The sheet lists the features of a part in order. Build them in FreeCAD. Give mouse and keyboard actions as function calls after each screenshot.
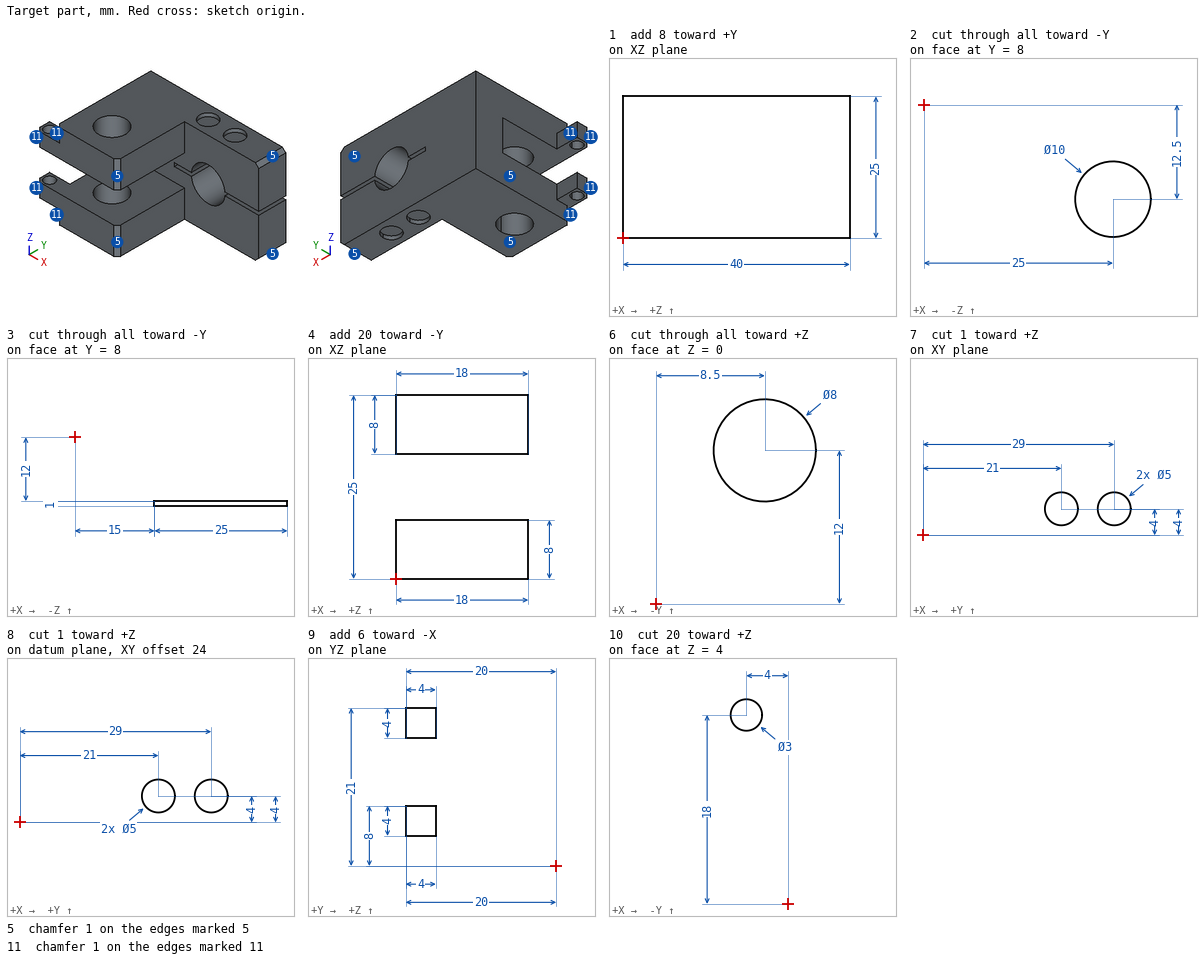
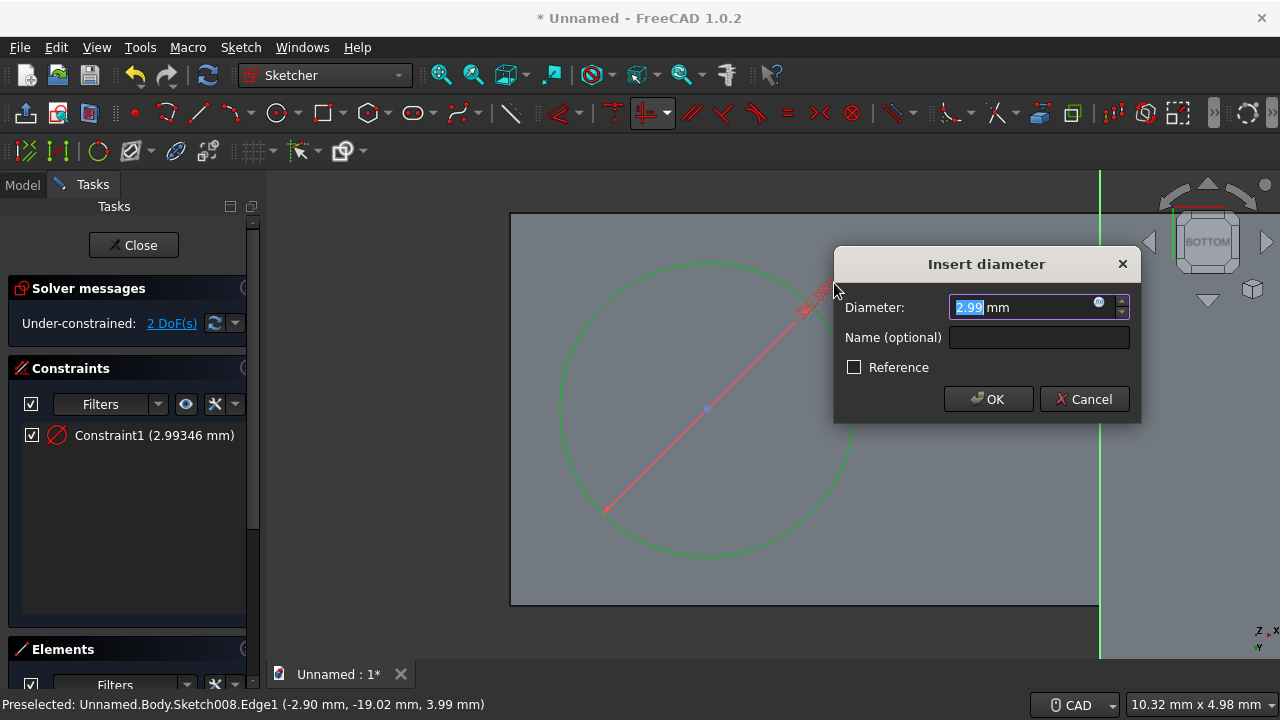
text(3)
key(Return)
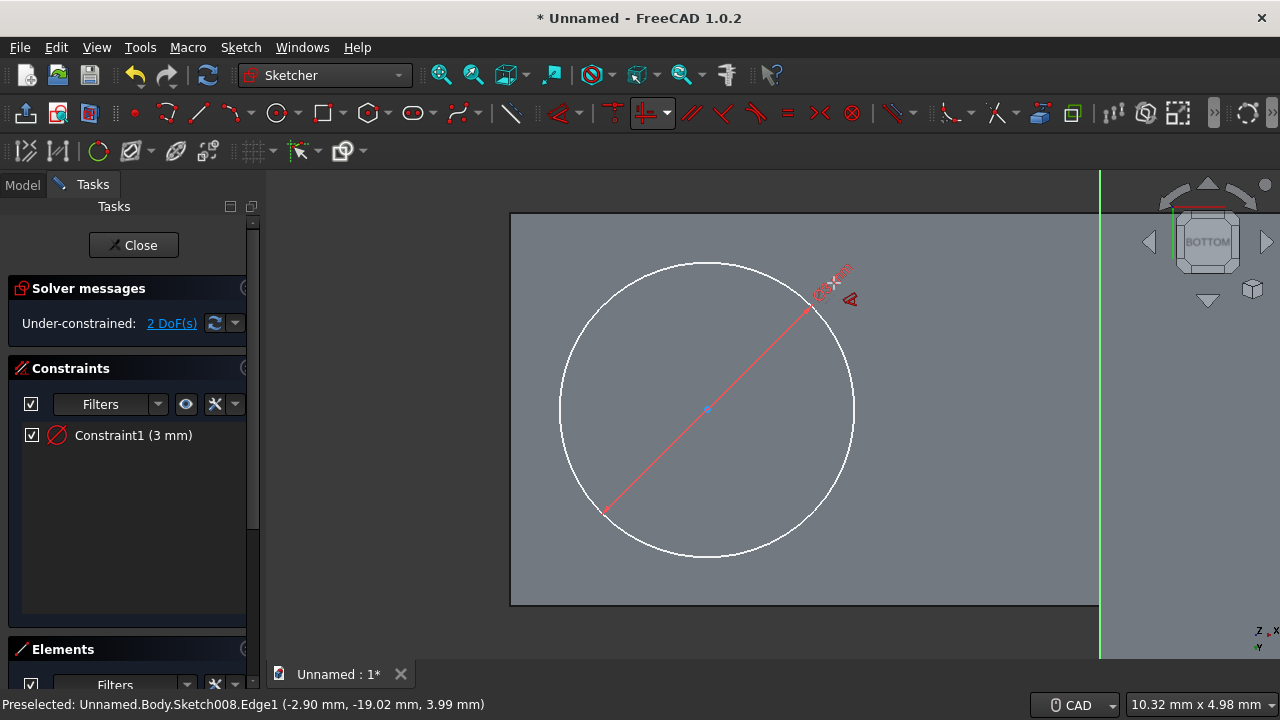
click(707, 410)
click(903, 376)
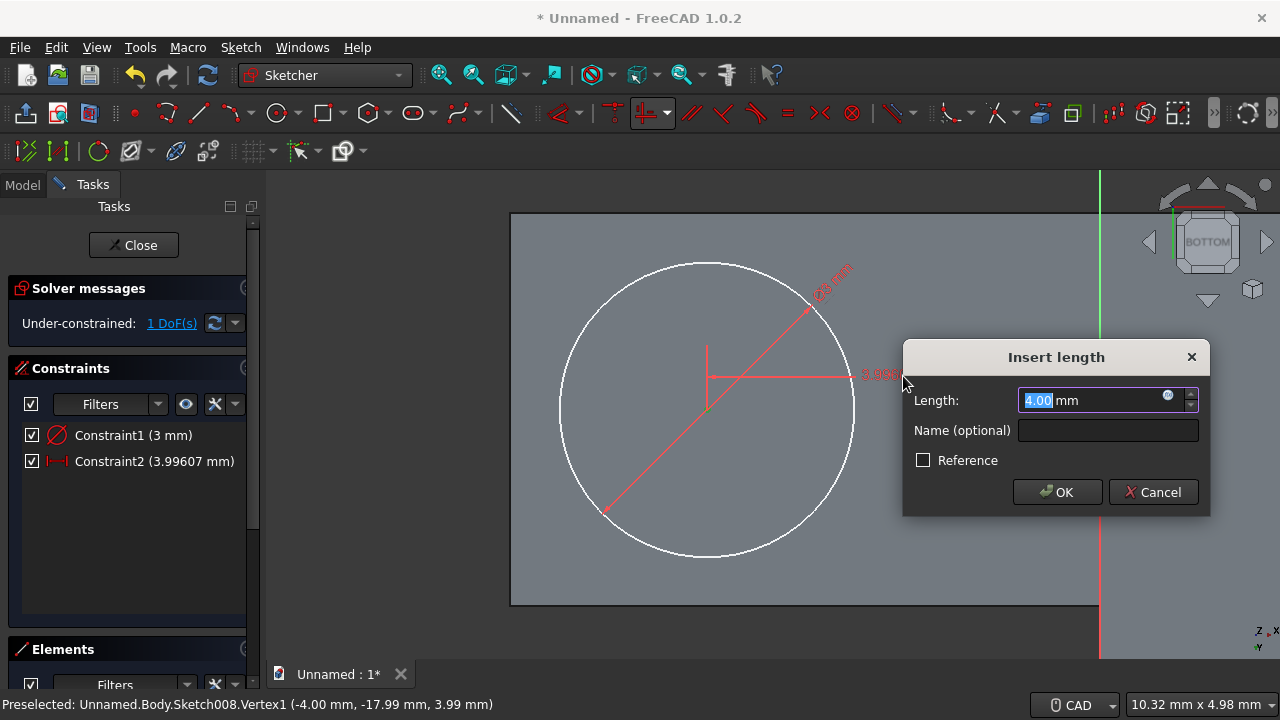
text(4)
key(Return)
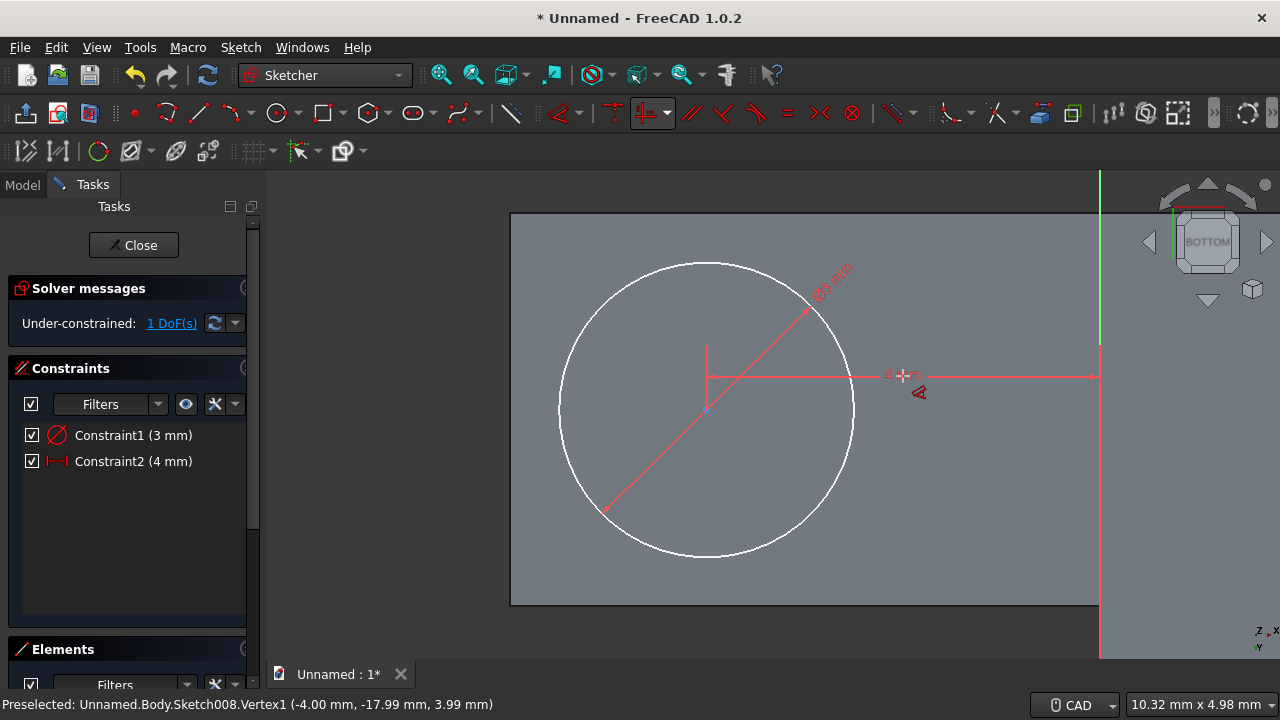
click(707, 410)
click(673, 521)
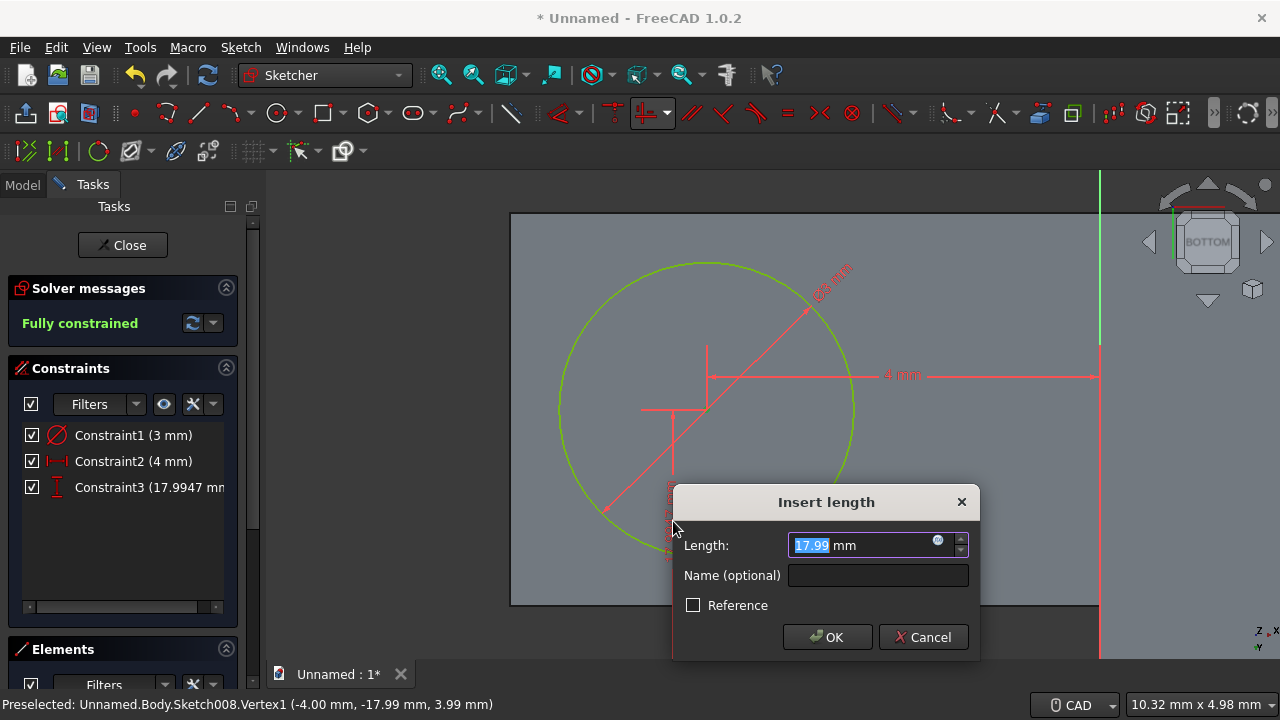
text(18)
key(Return)
key(Escape)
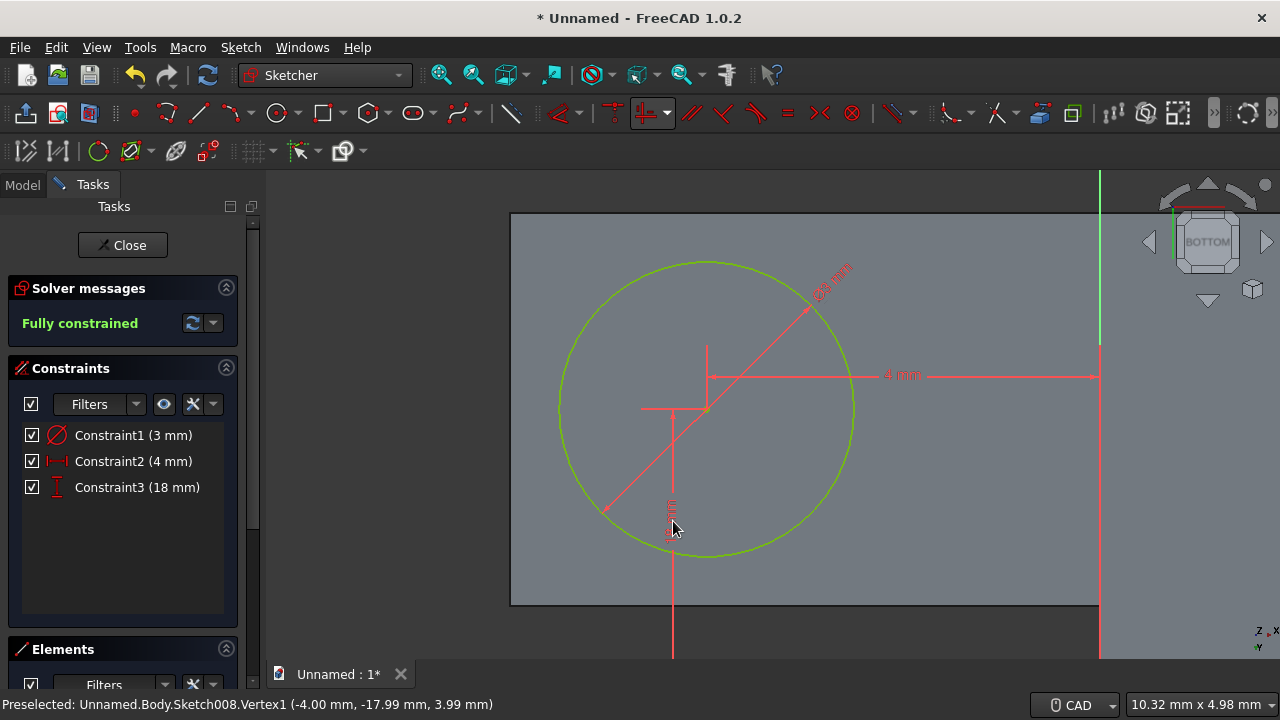
click(123, 245)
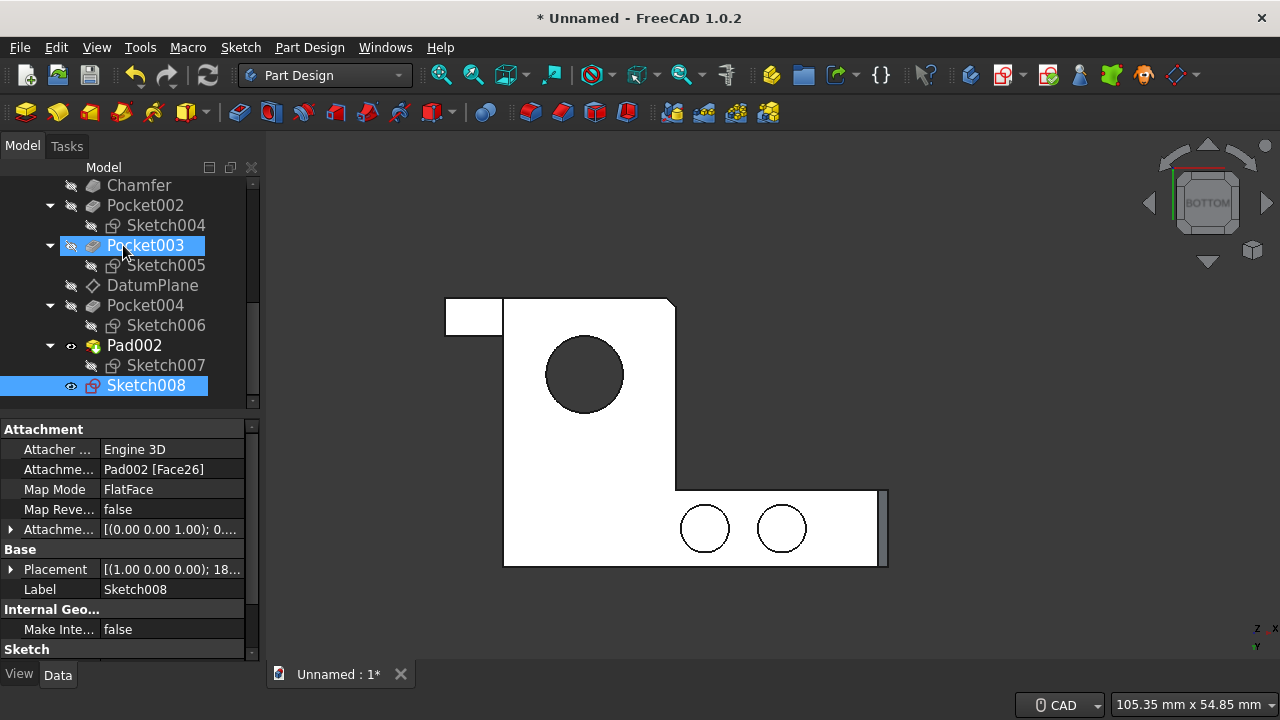
click(240, 112)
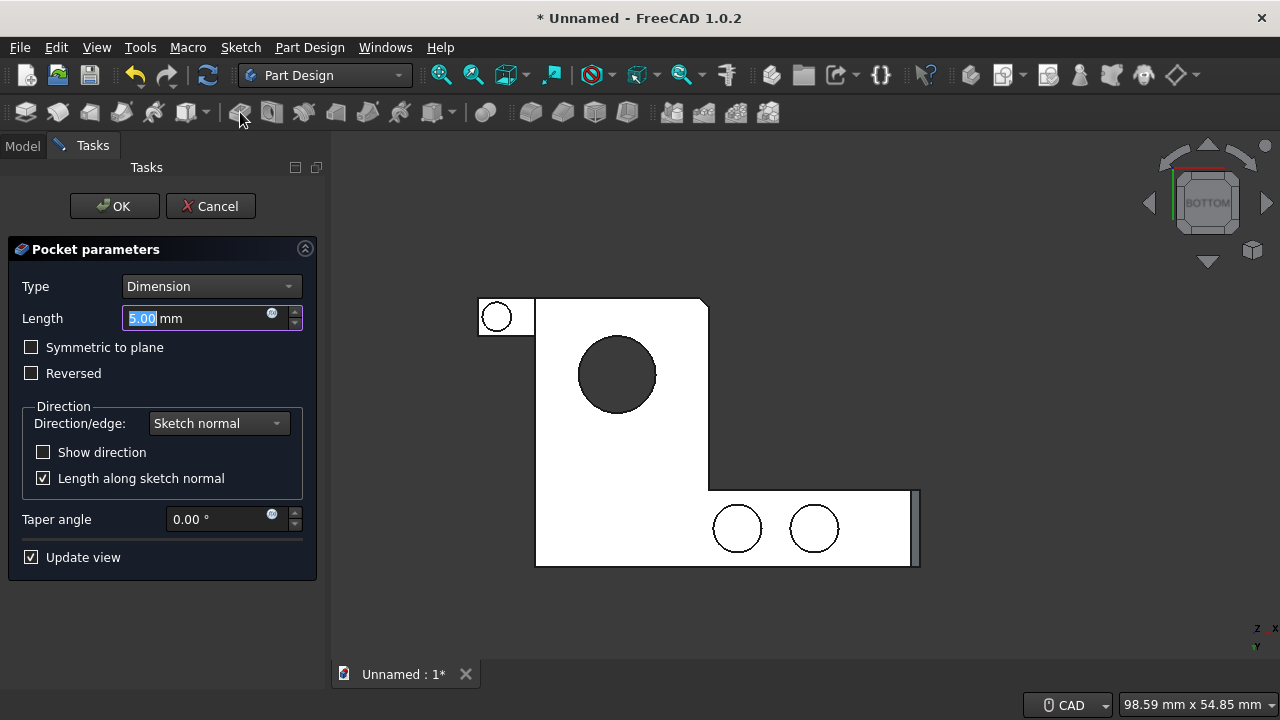
text(20)
key(Tab)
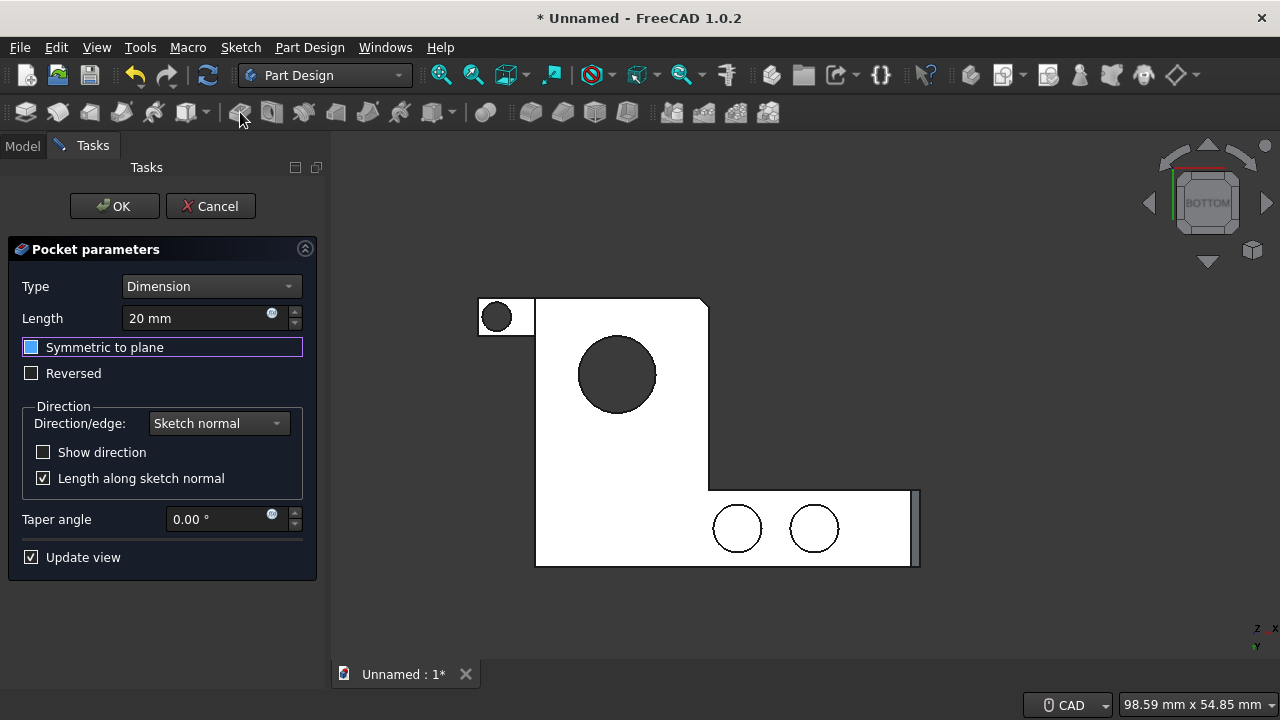
click(115, 206)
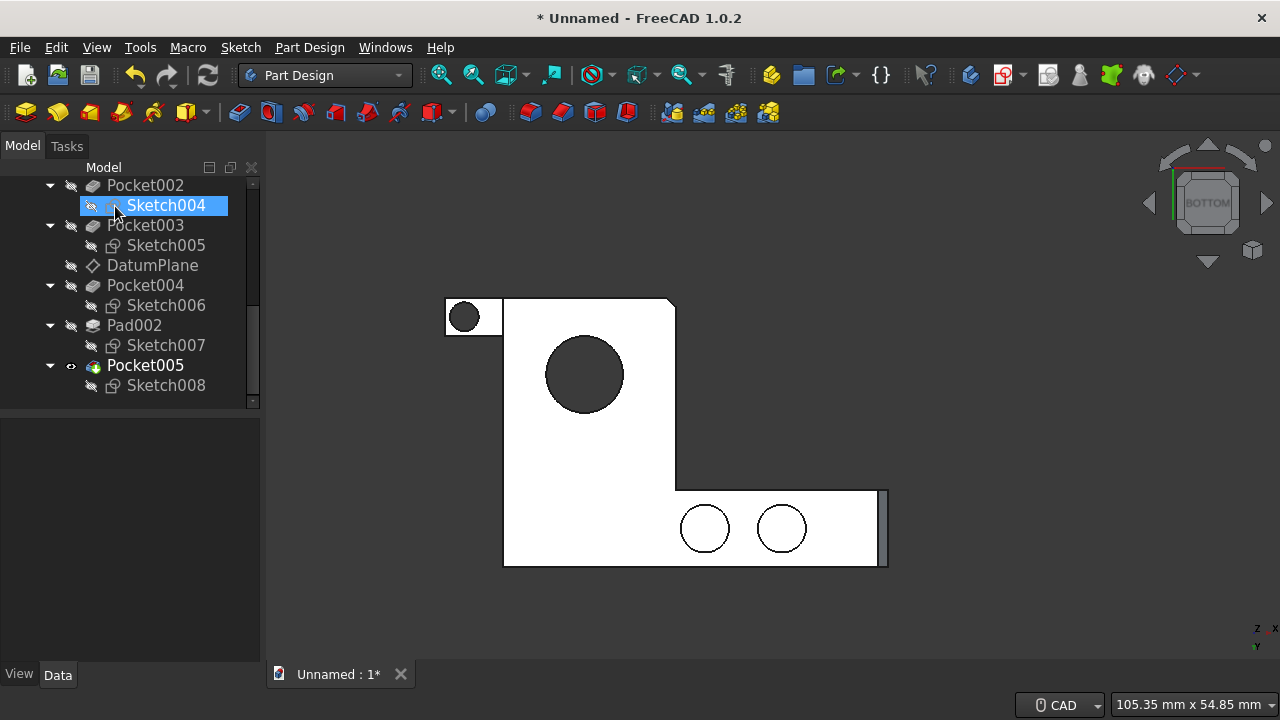
key(0)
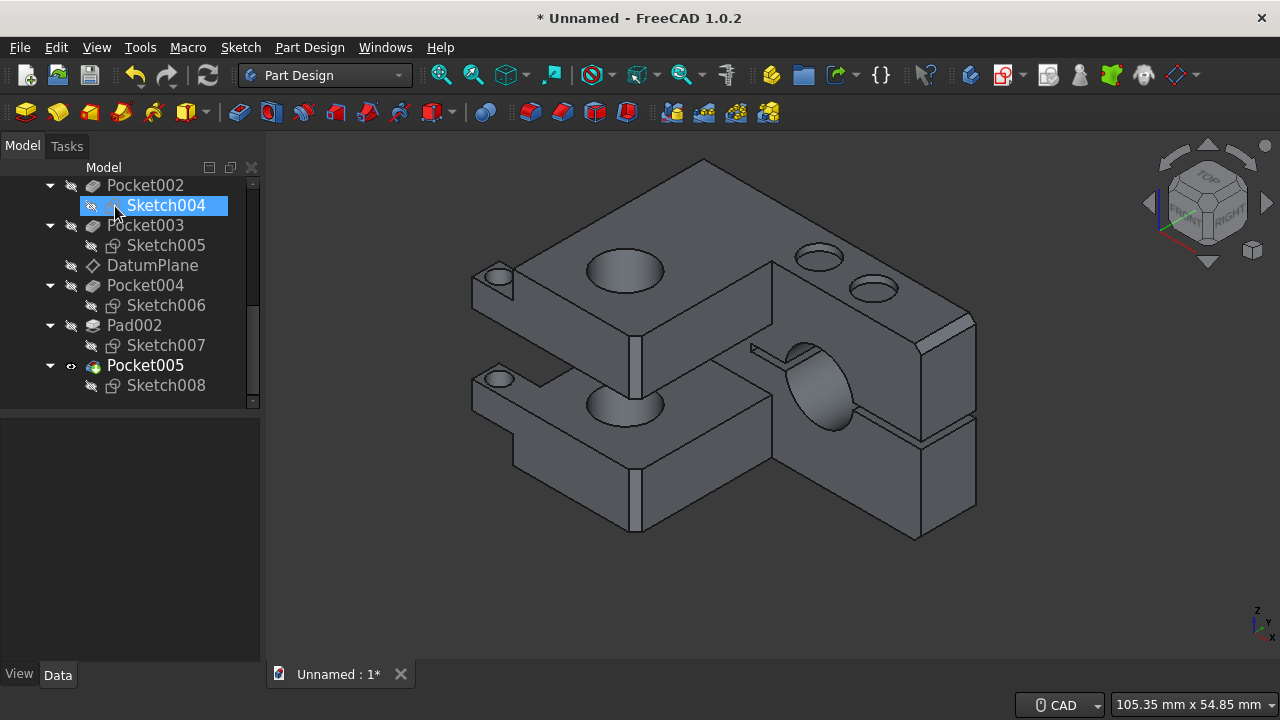
key(2)